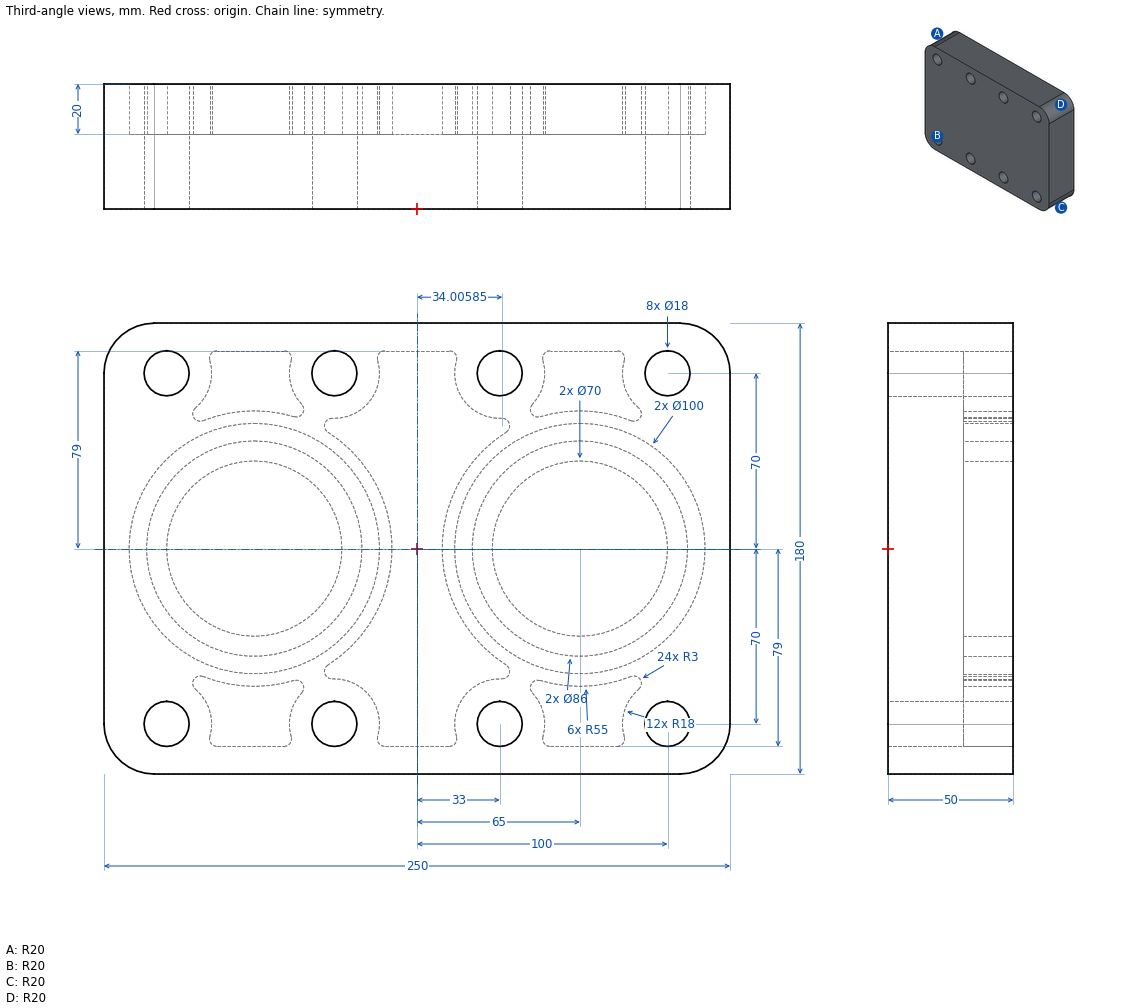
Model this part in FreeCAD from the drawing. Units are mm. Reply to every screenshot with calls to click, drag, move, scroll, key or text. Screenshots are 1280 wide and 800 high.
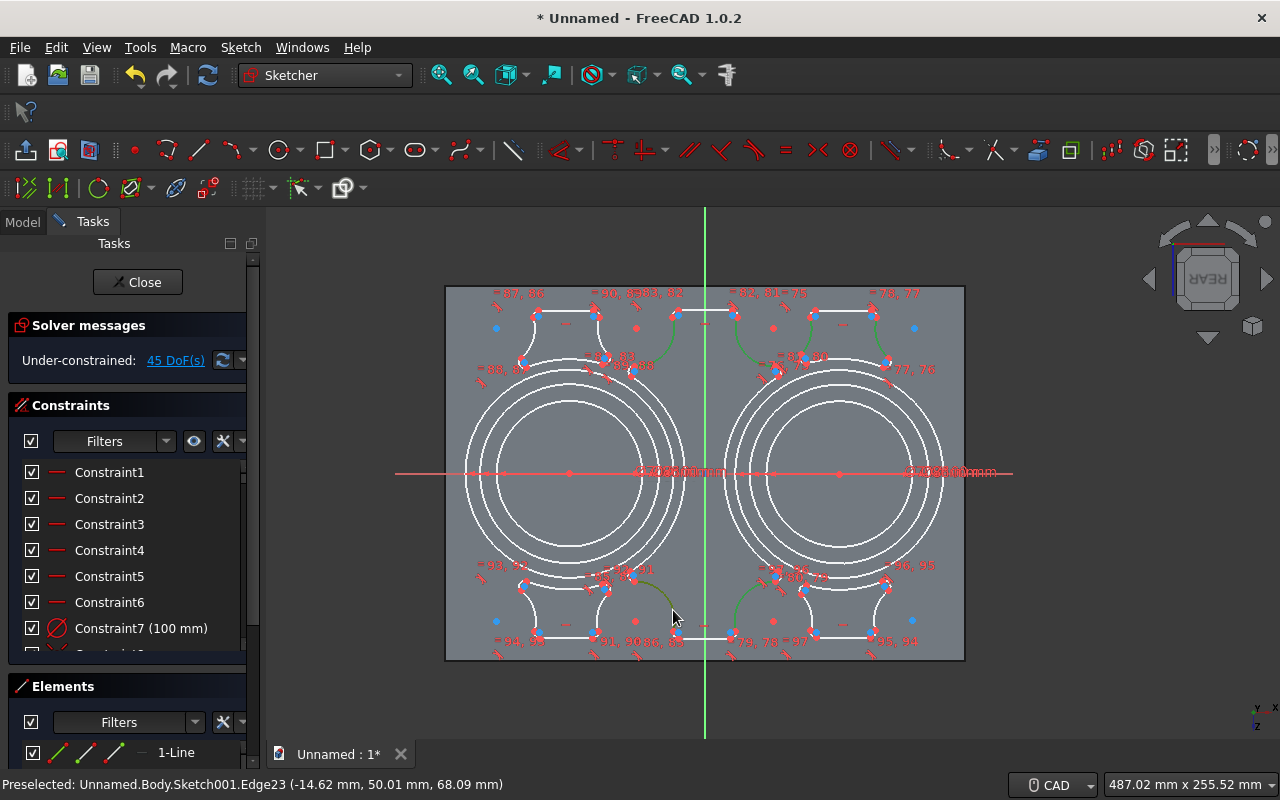
click(530, 348)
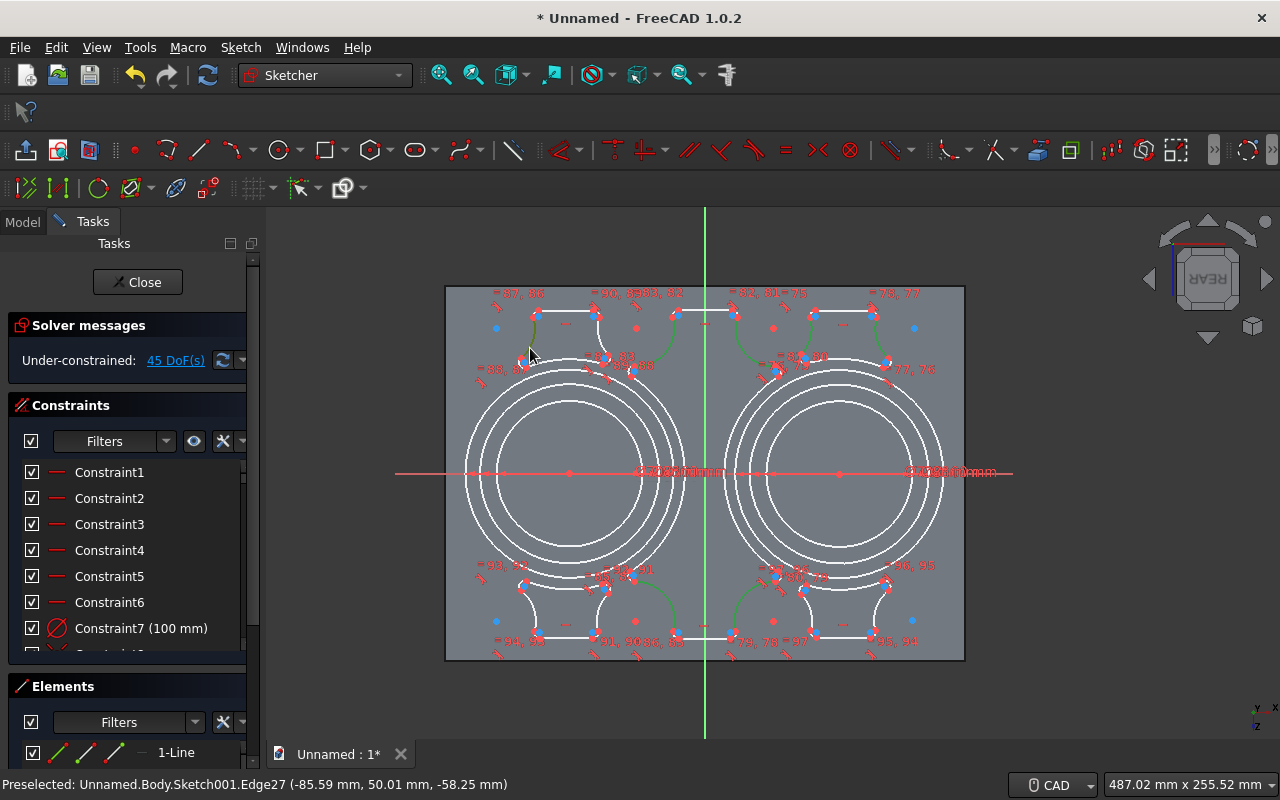
click(598, 330)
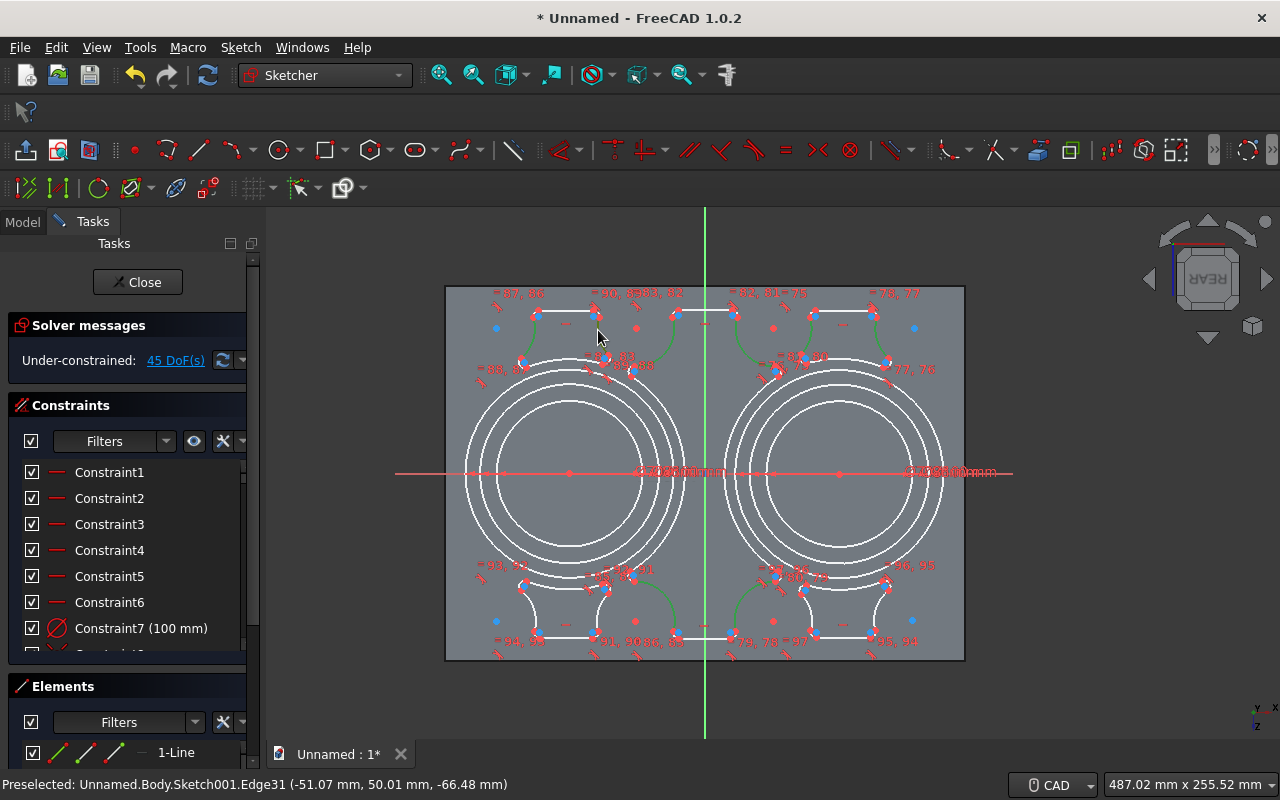
click(601, 604)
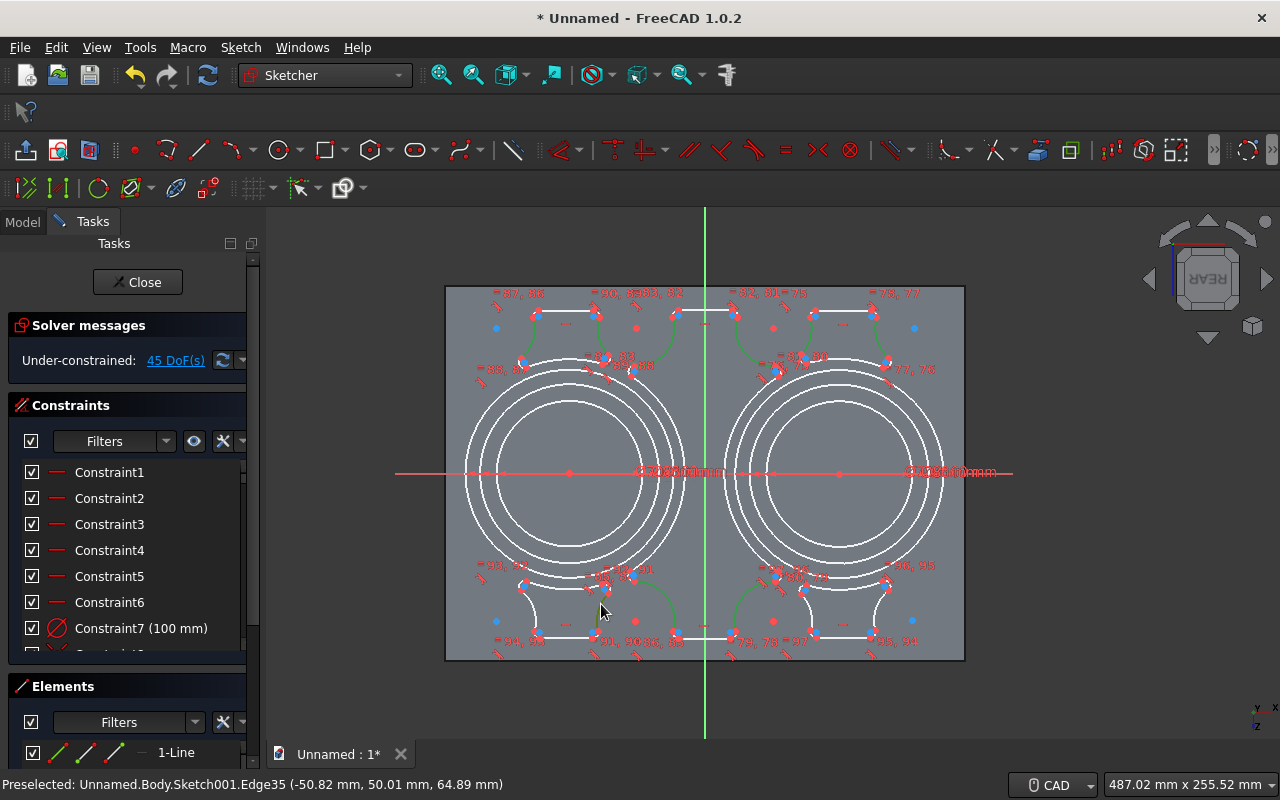
click(536, 618)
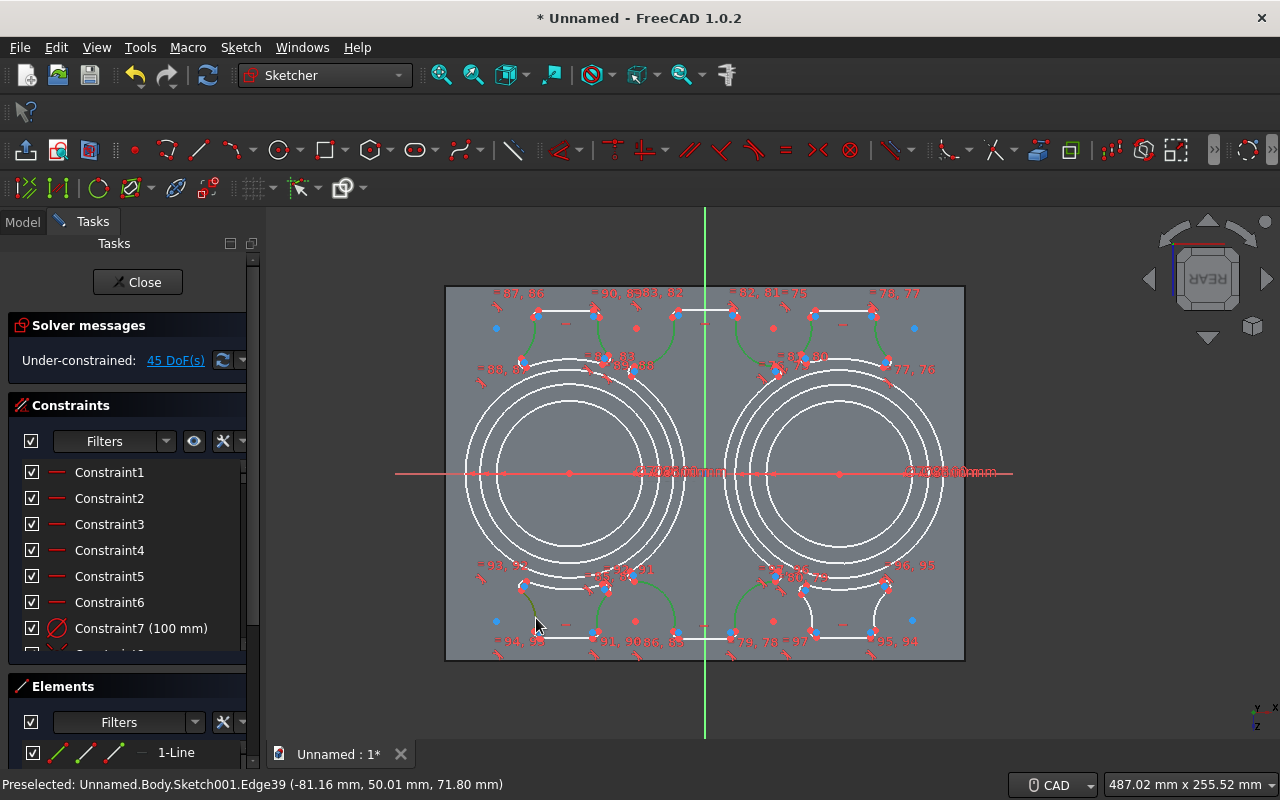
click(880, 601)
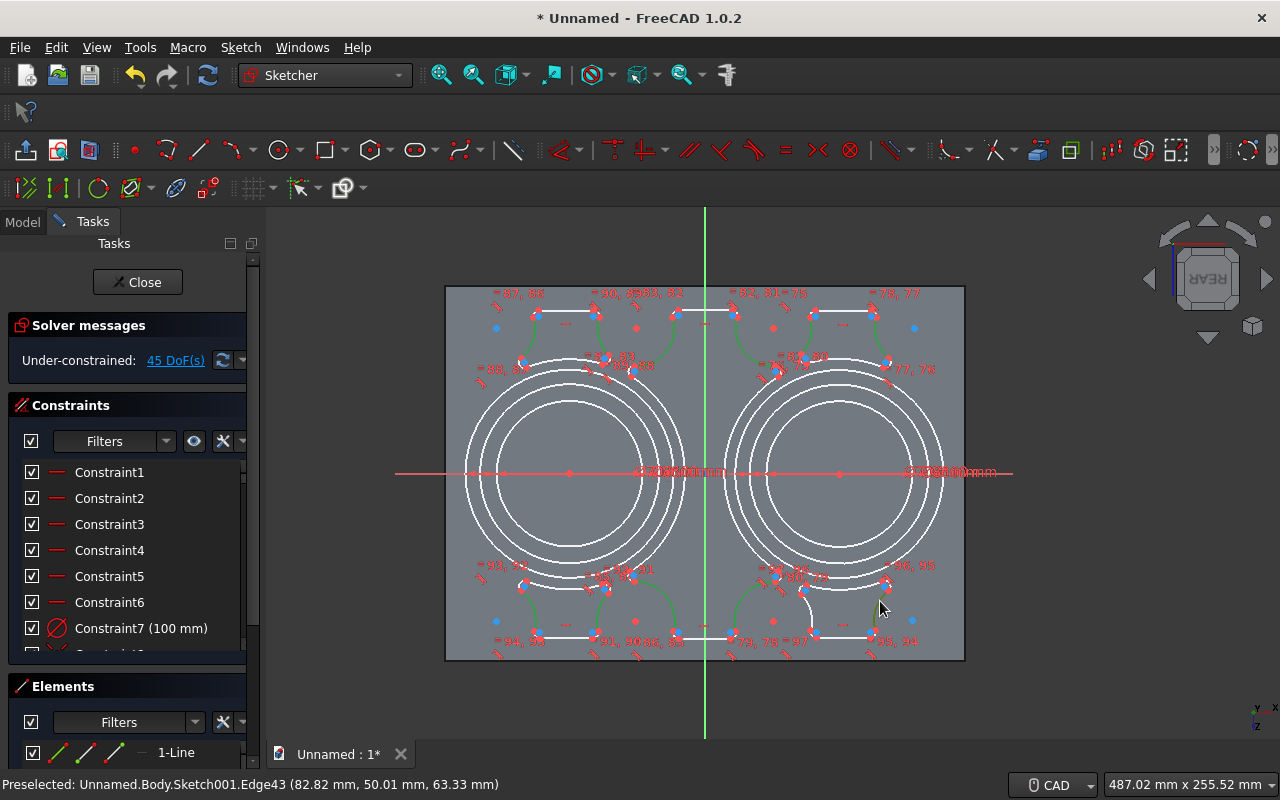
click(812, 619)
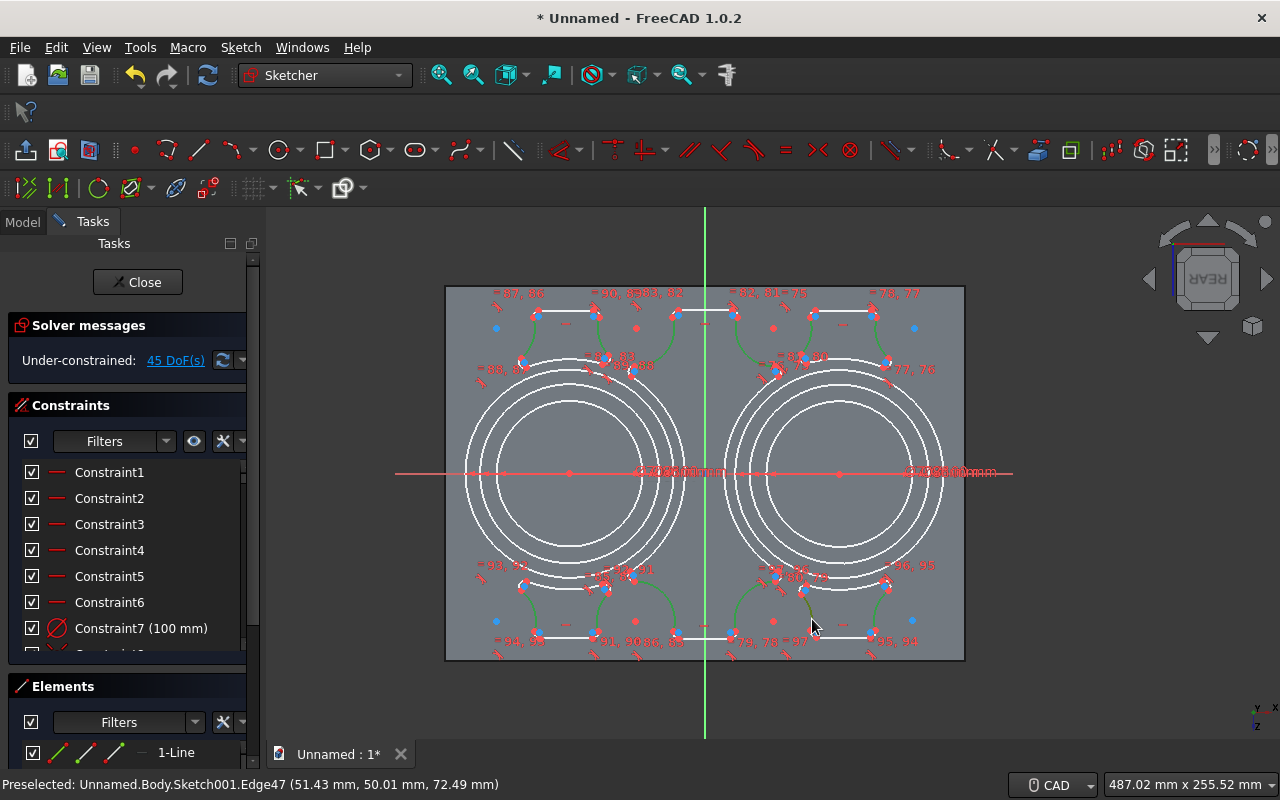
click(786, 150)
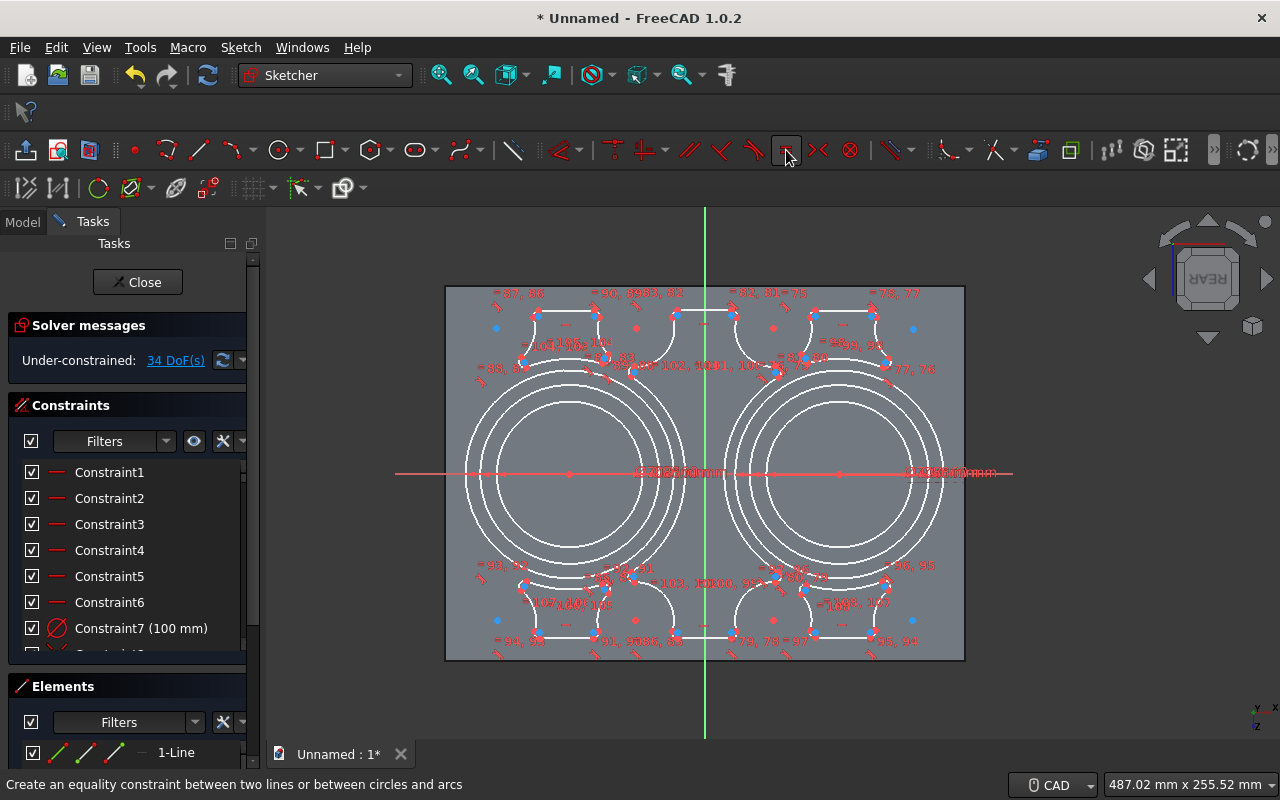
click(861, 361)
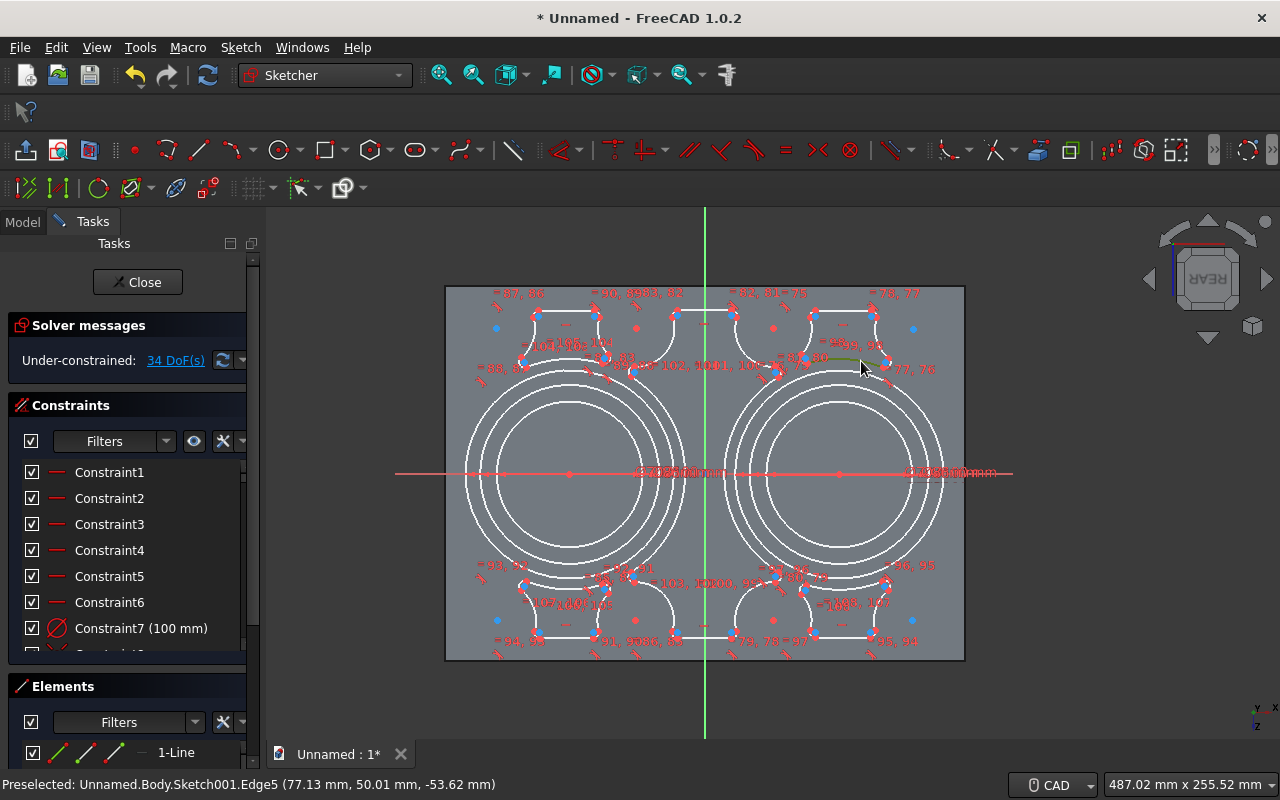
scroll(734, 429, up, 2)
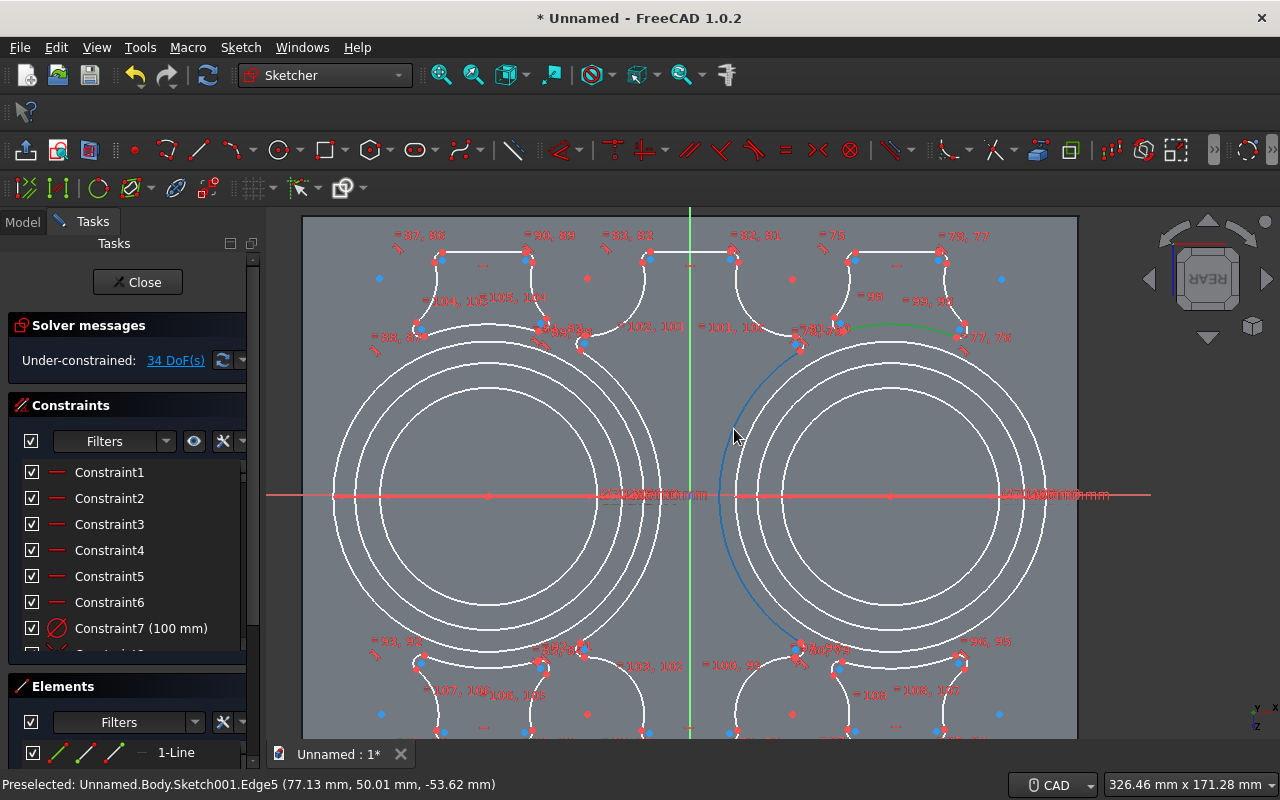
click(733, 429)